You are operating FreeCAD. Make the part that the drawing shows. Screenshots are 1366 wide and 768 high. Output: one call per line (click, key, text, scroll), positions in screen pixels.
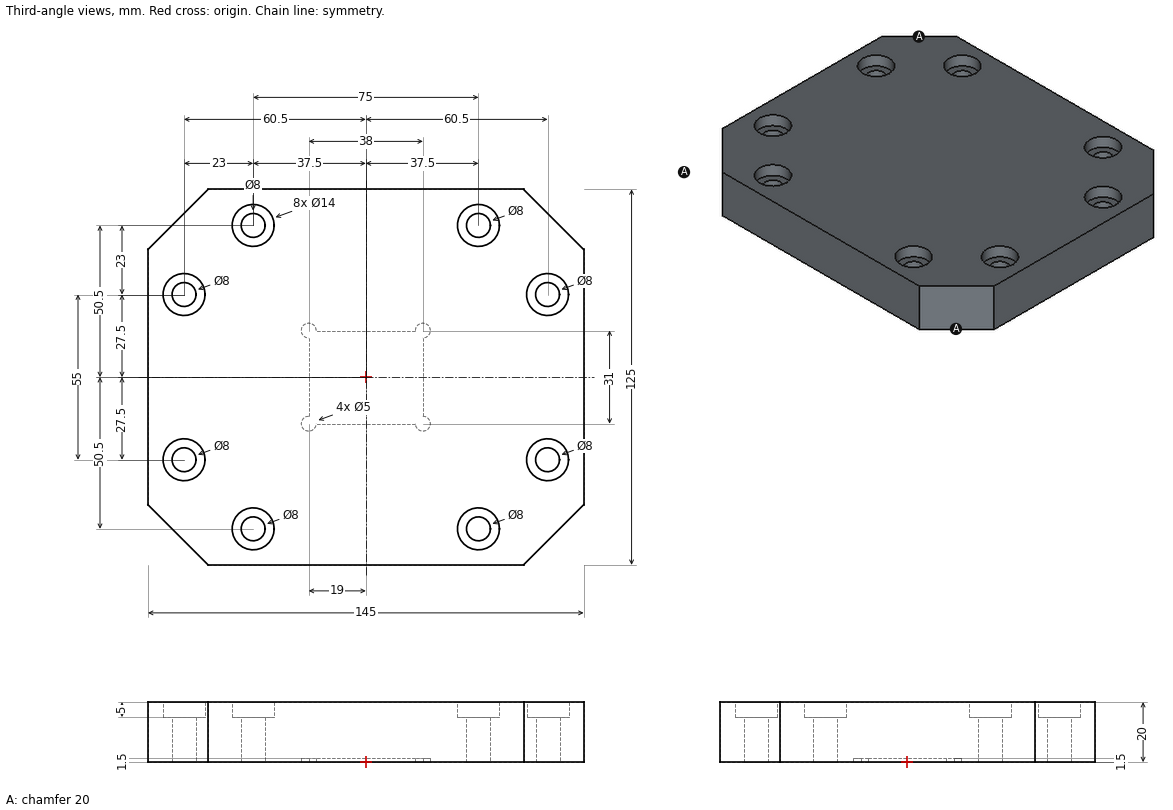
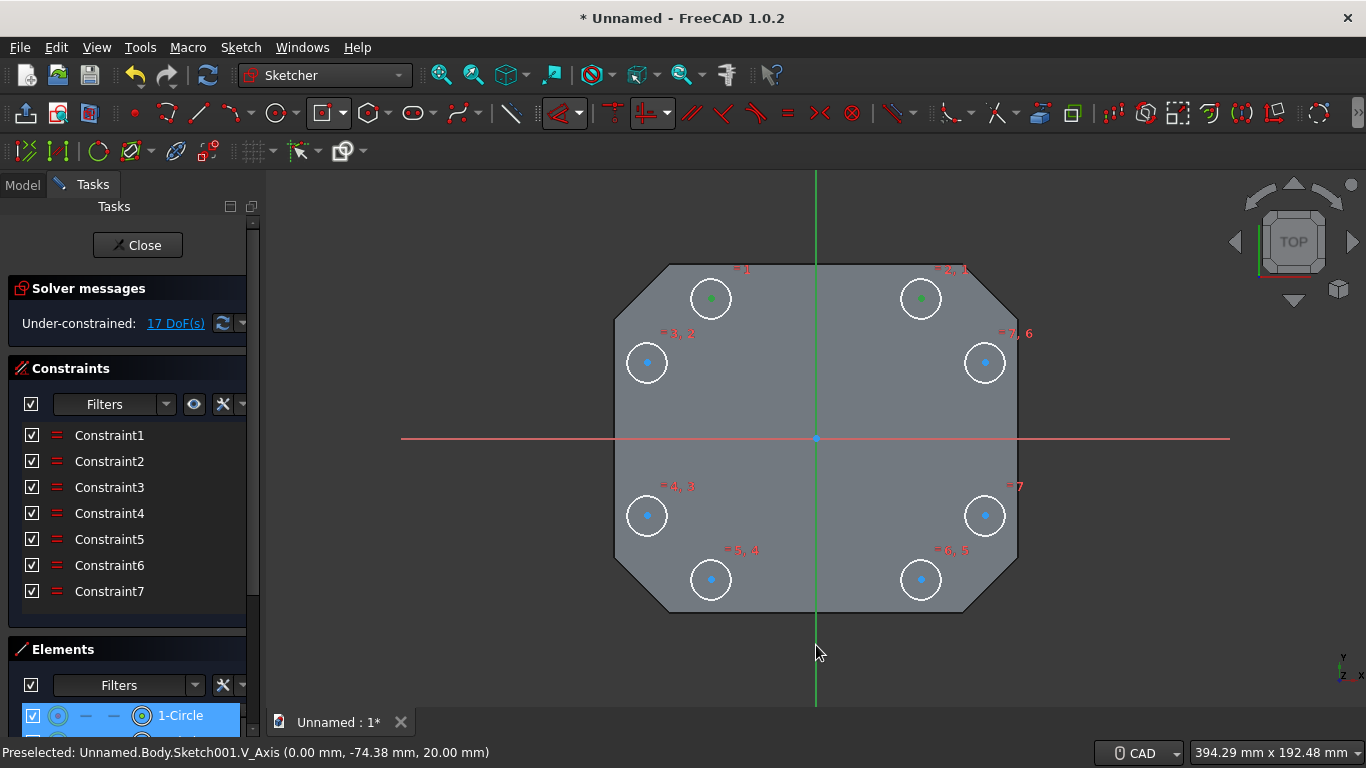
click(820, 114)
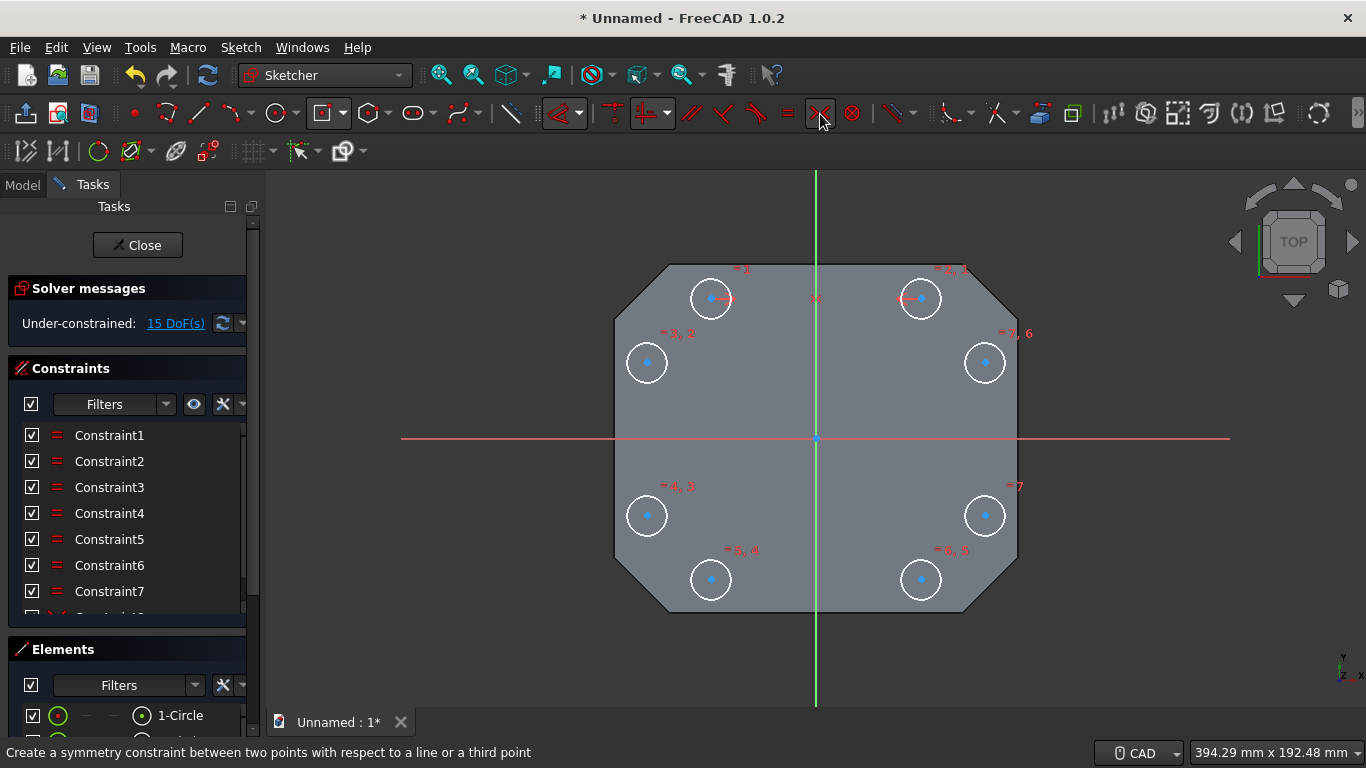
click(647, 363)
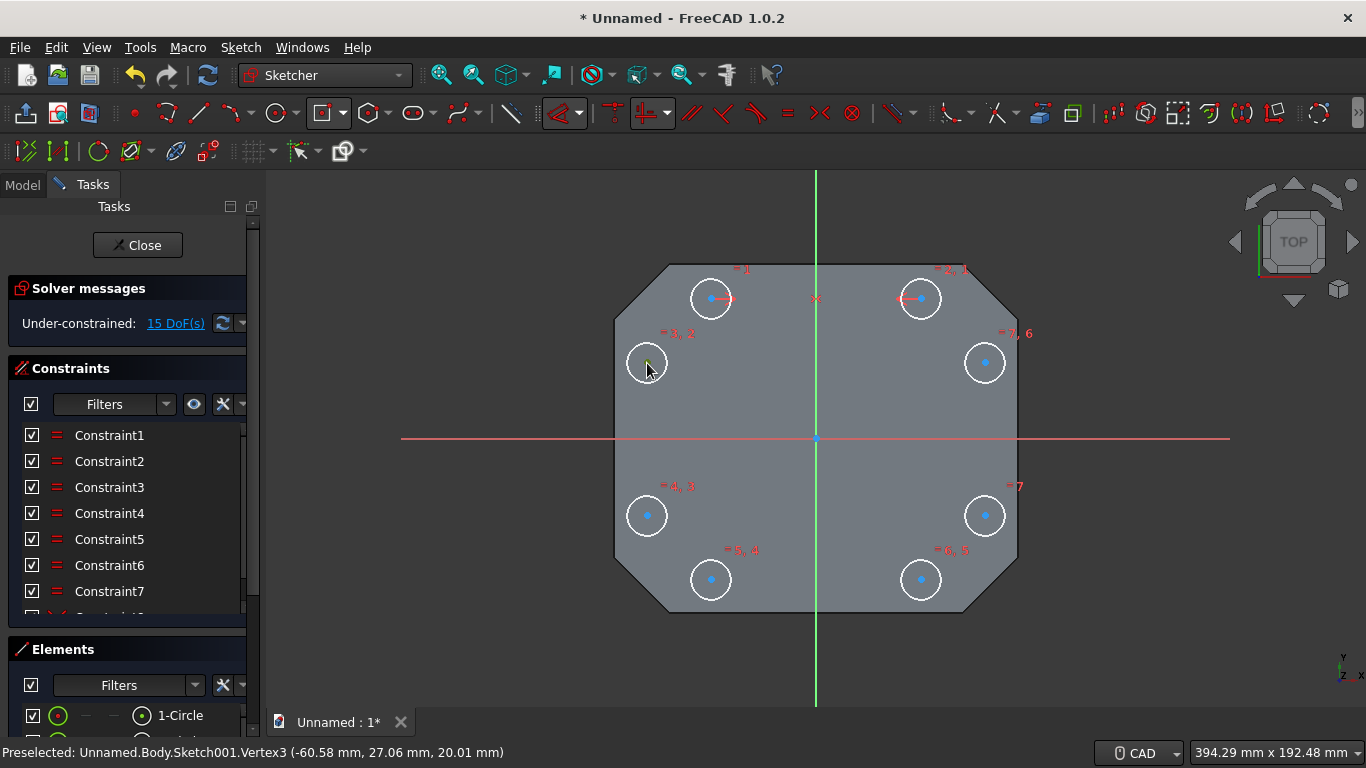
click(647, 516)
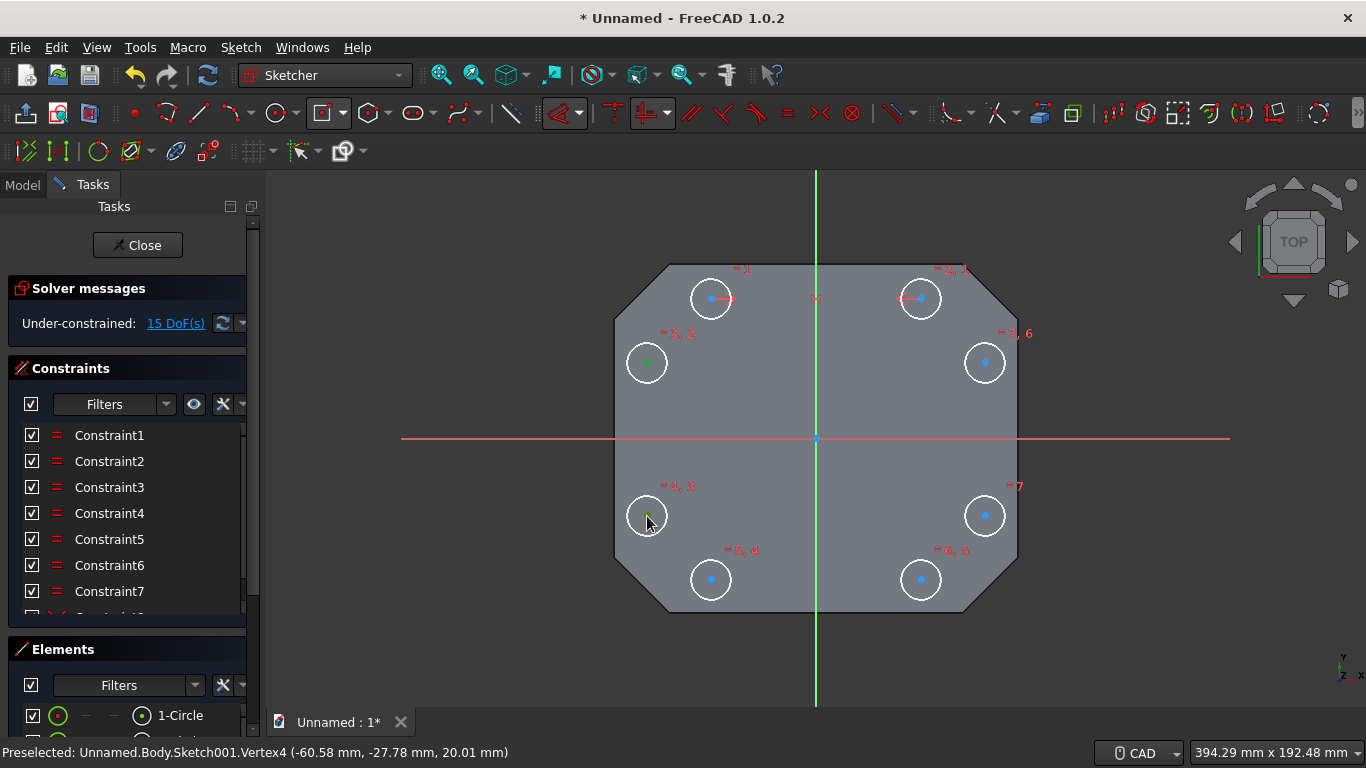
click(424, 438)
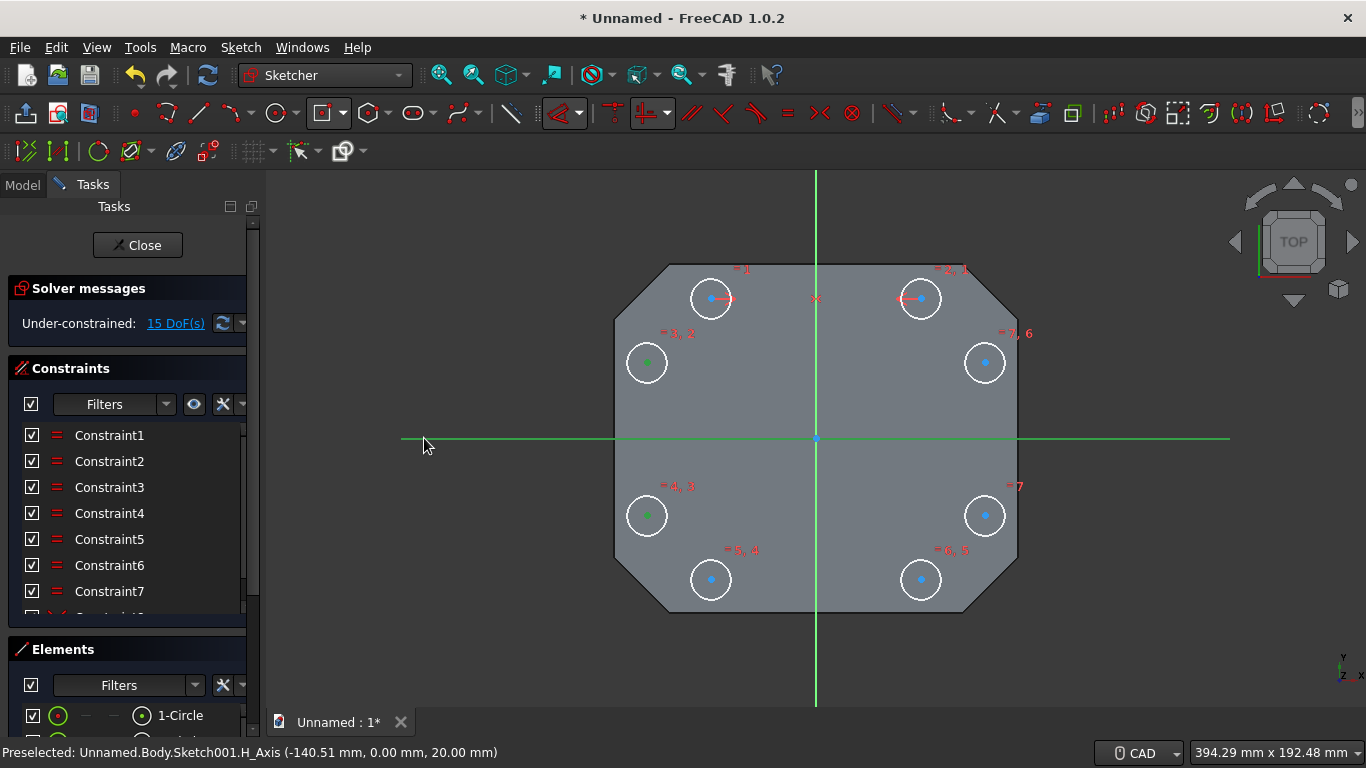
key(s)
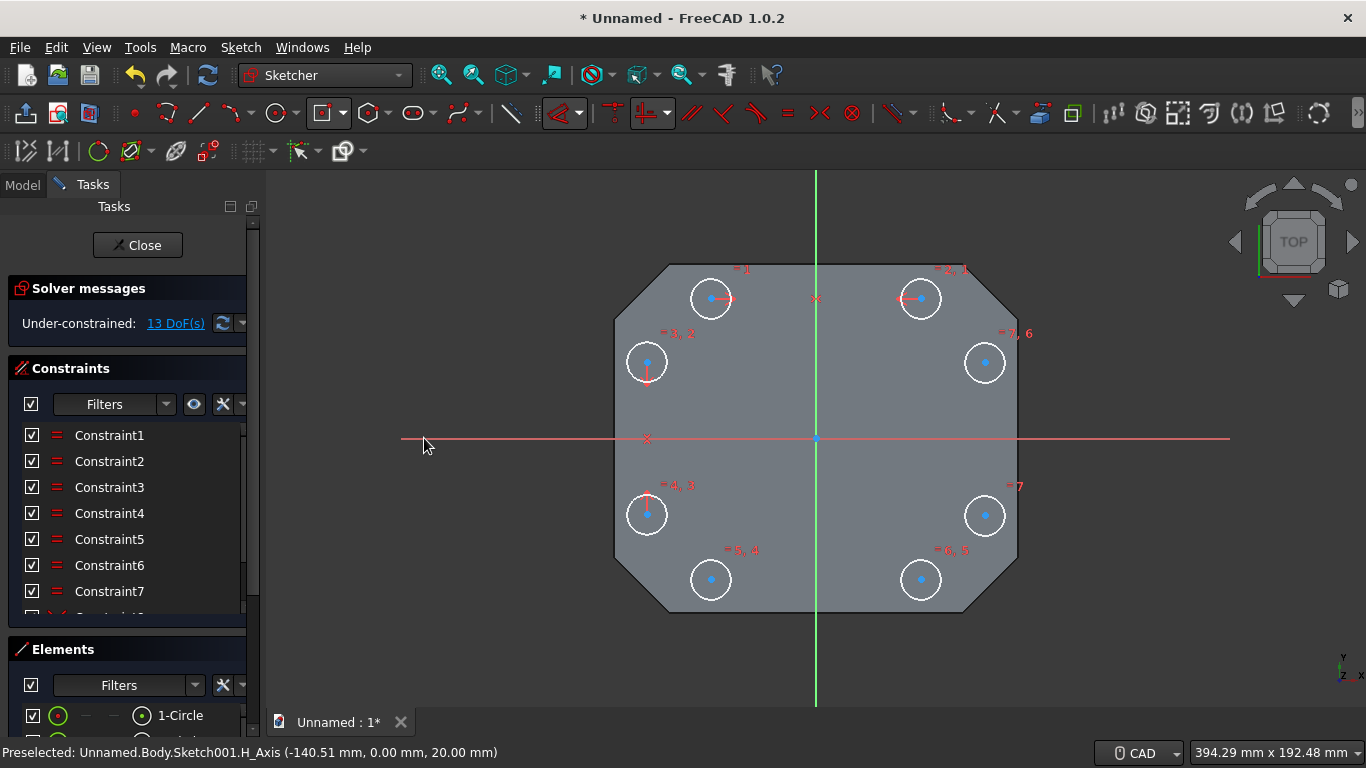
click(711, 299)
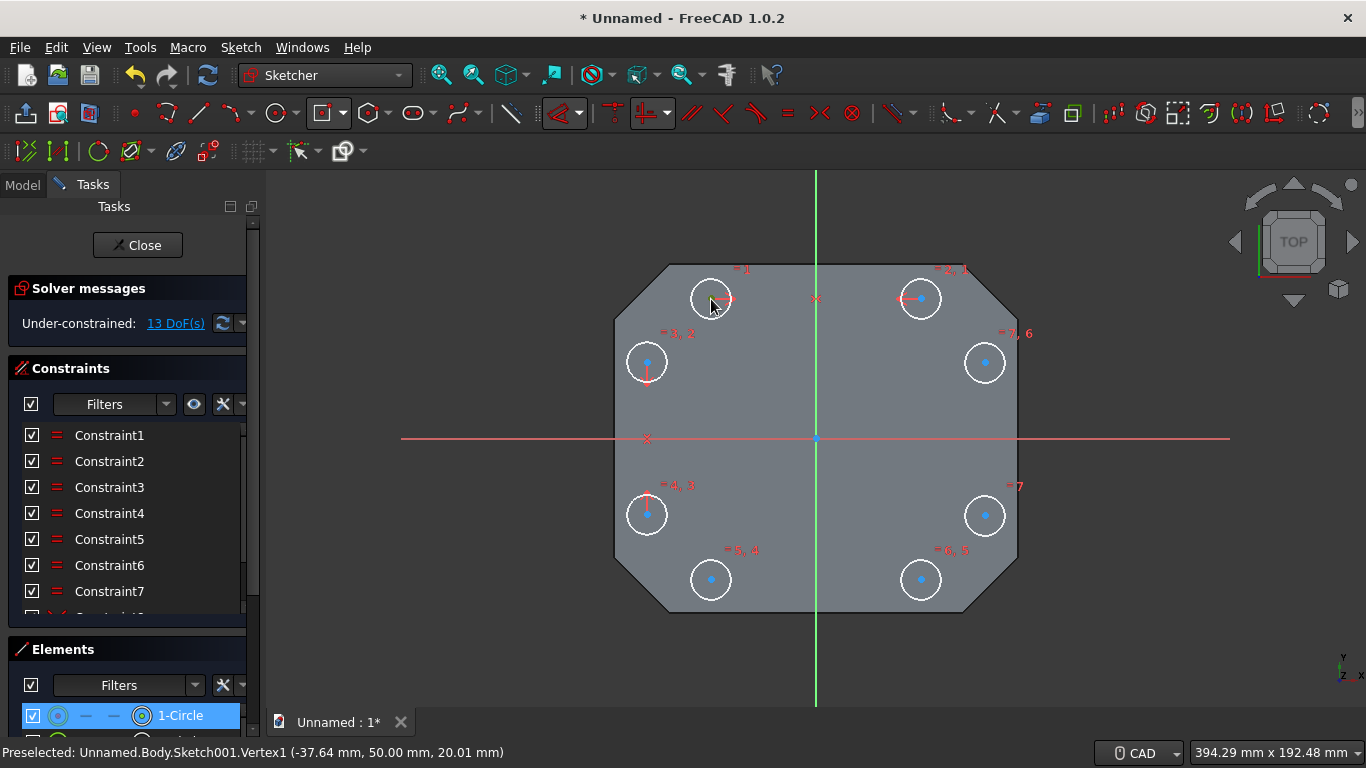
click(711, 580)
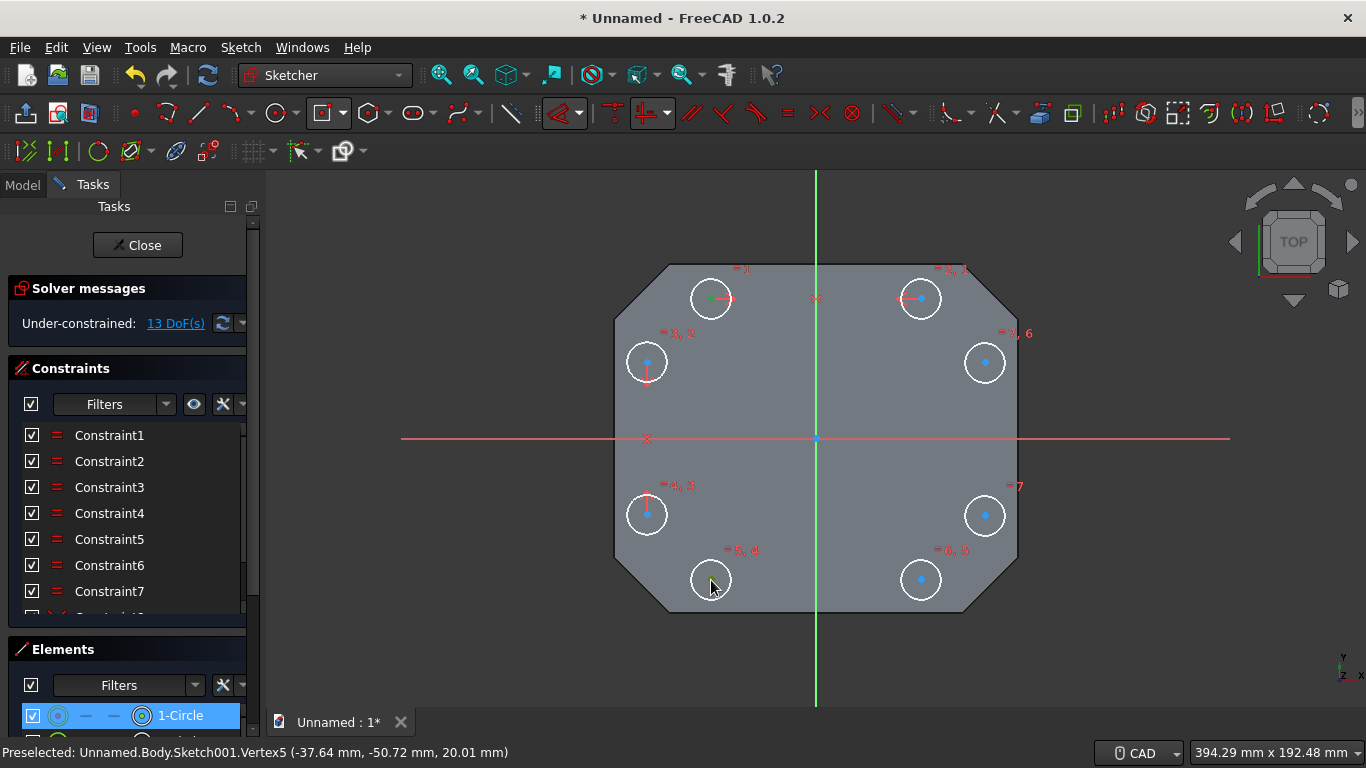
click(424, 438)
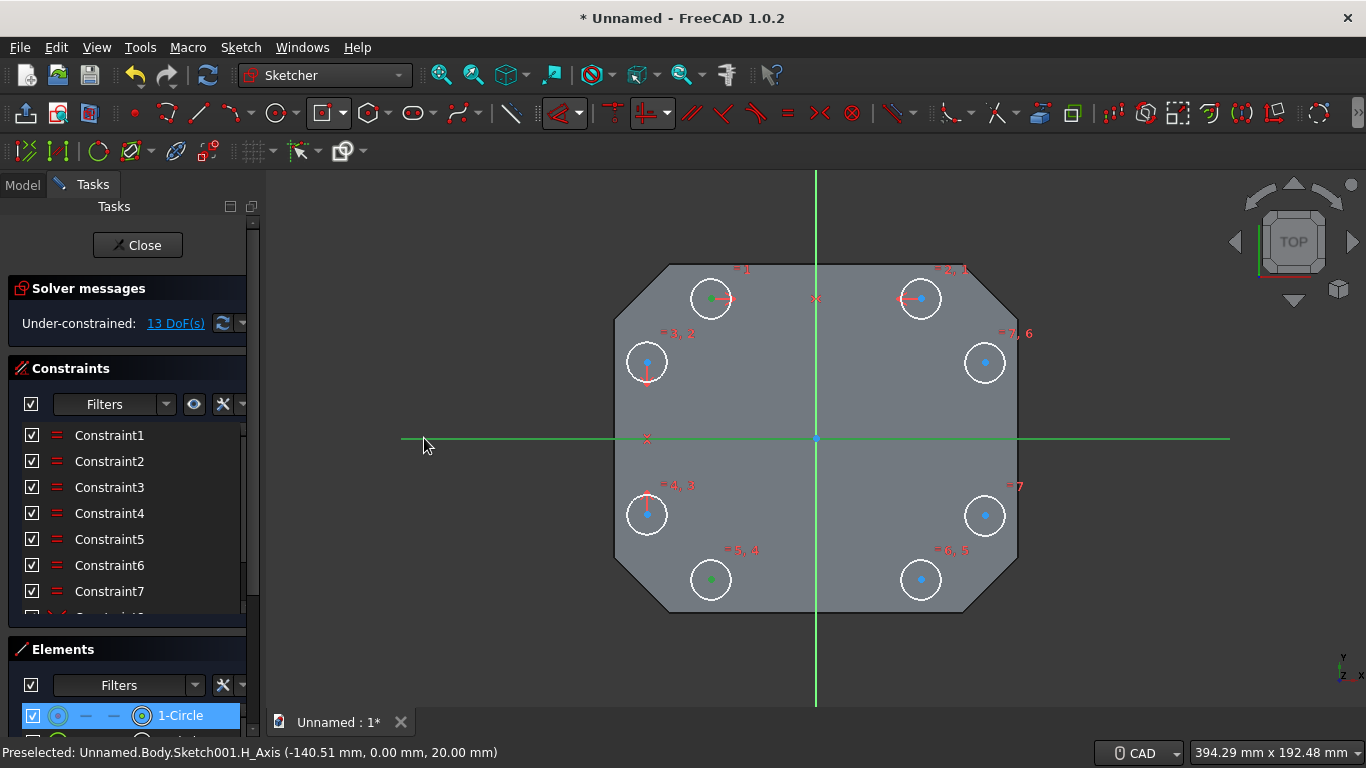
click(820, 114)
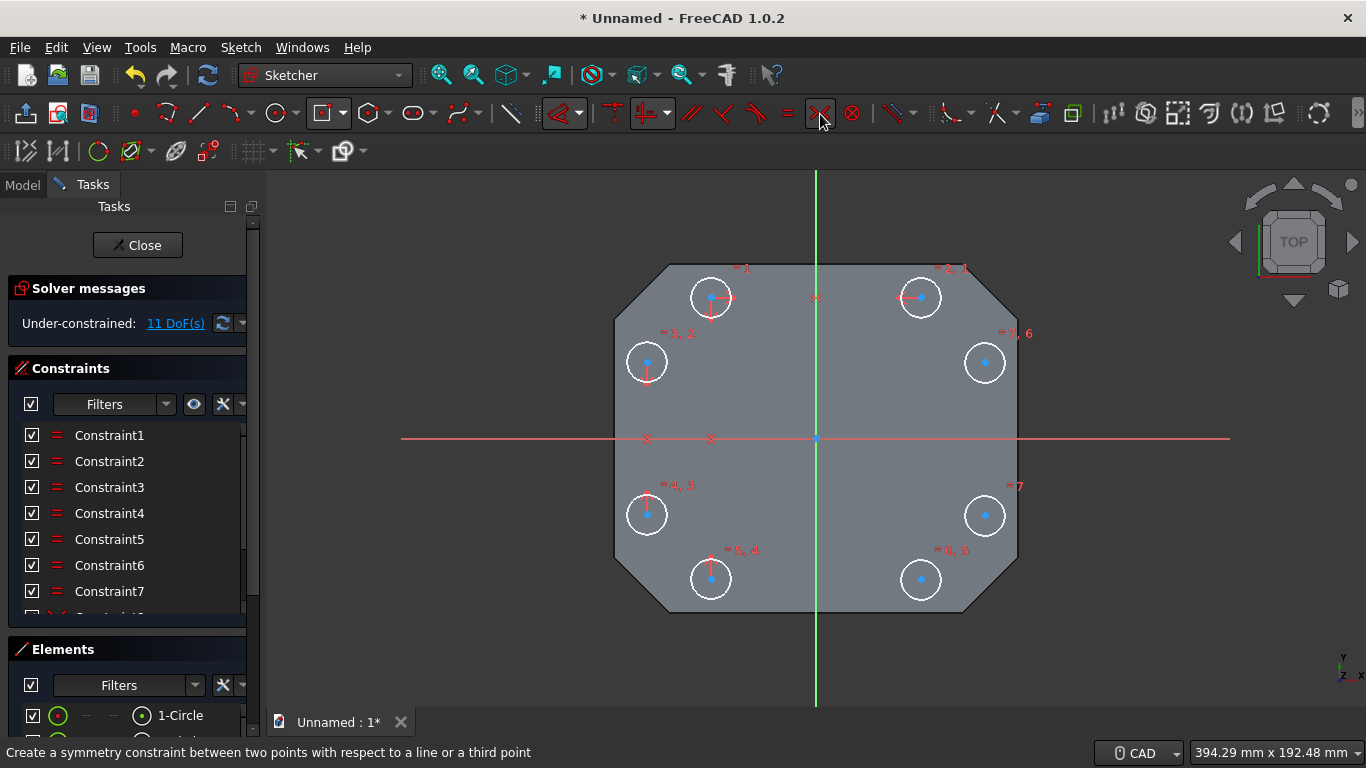
click(921, 298)